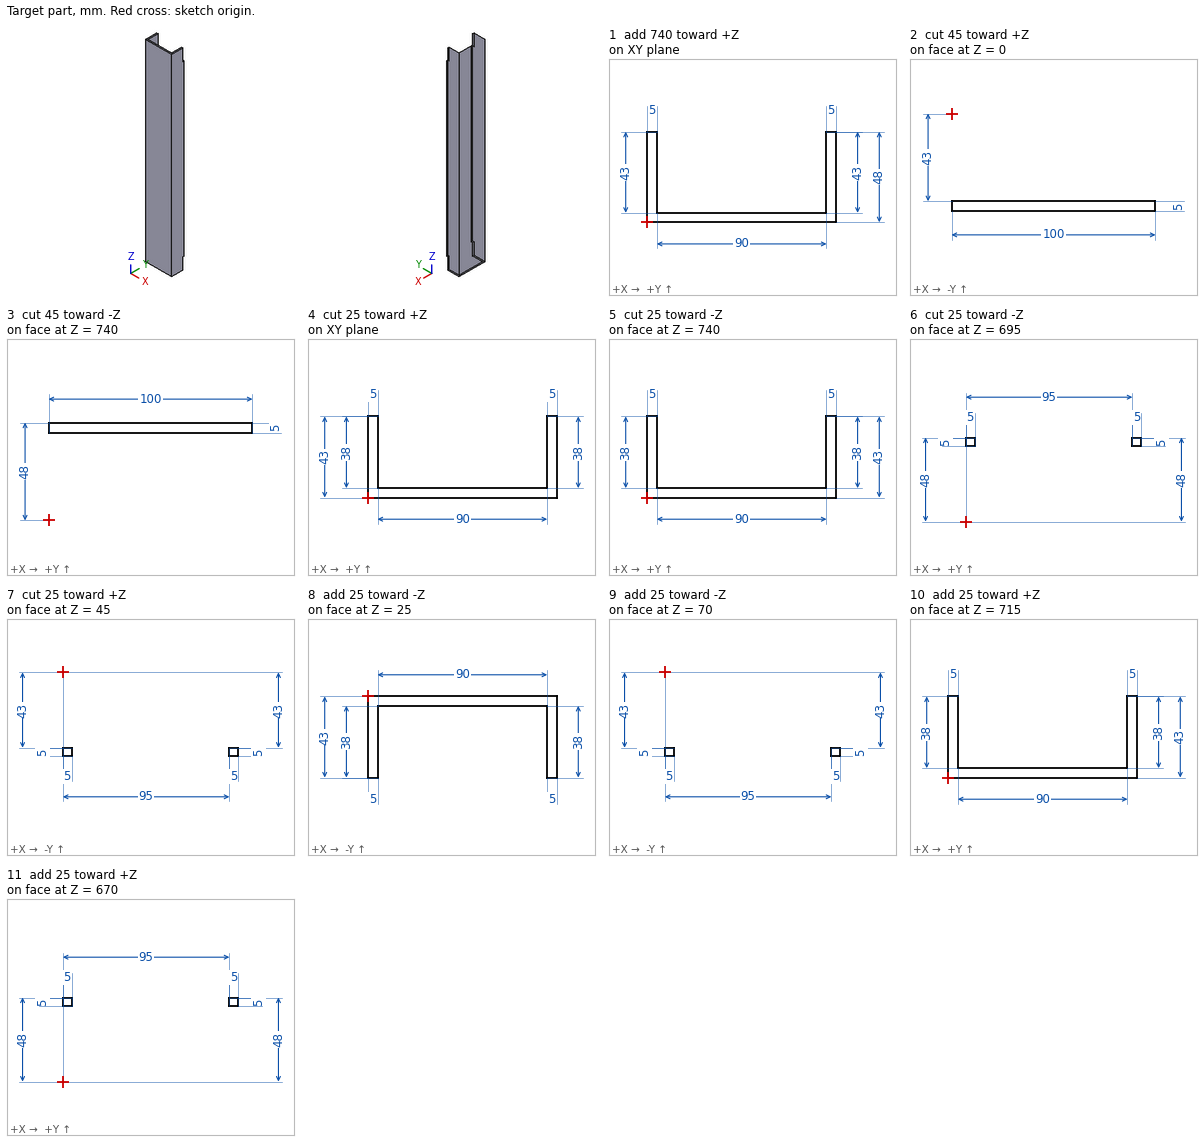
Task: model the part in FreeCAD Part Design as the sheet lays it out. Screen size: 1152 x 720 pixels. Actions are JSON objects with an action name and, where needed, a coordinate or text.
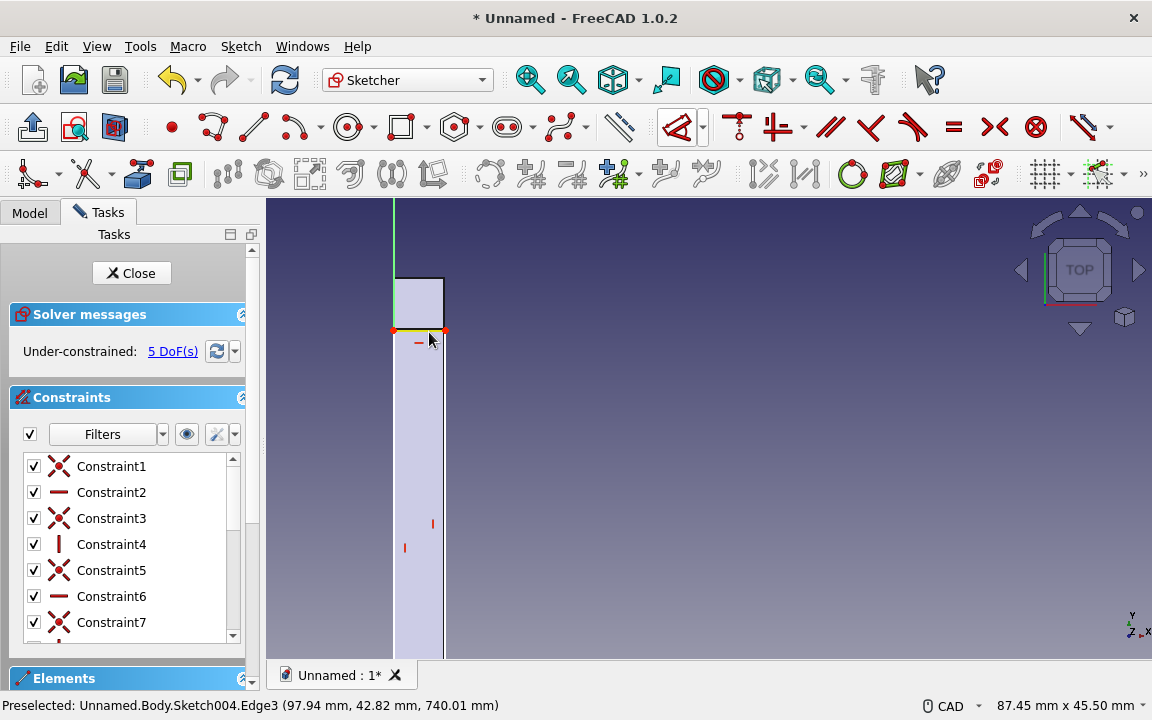
{"action": "left_click", "coordinate": [430, 331]}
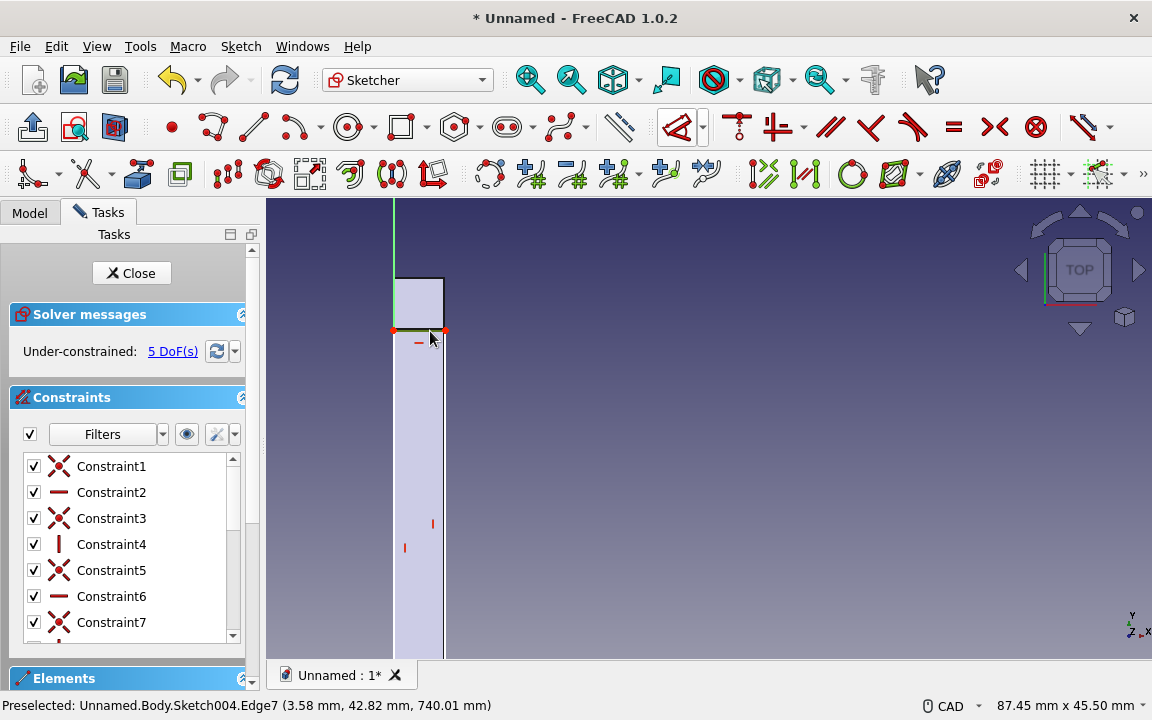
{"action": "left_click", "coordinate": [702, 128]}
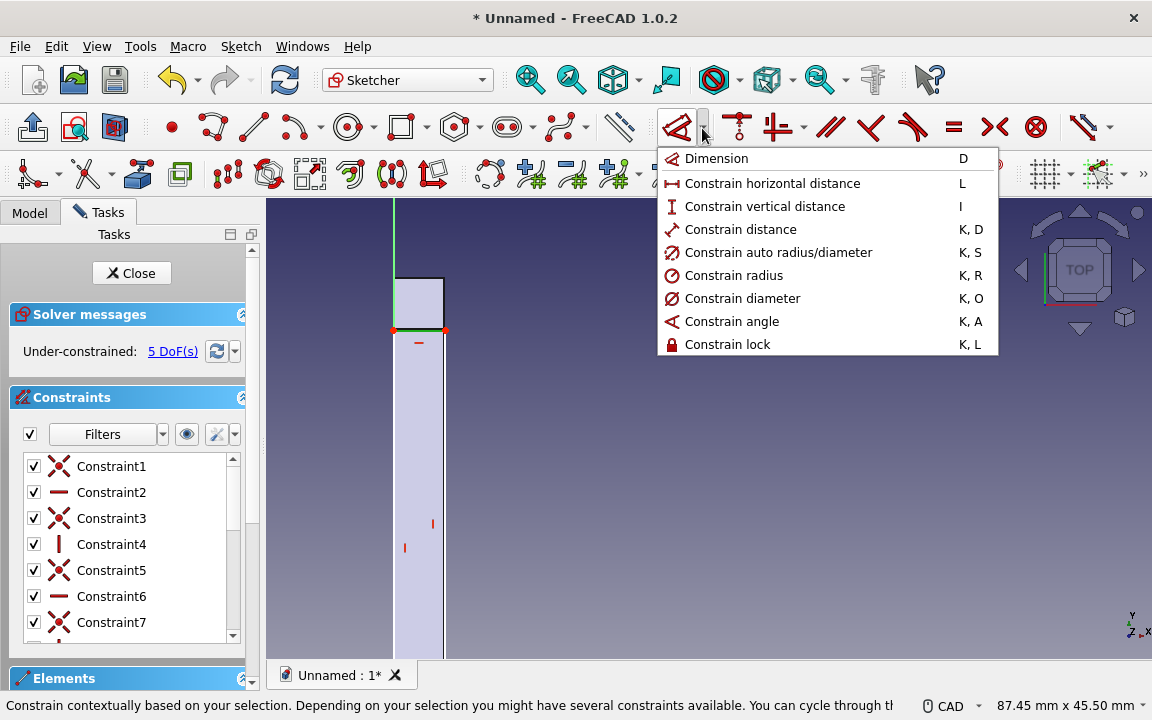
{"action": "left_click", "coordinate": [828, 184]}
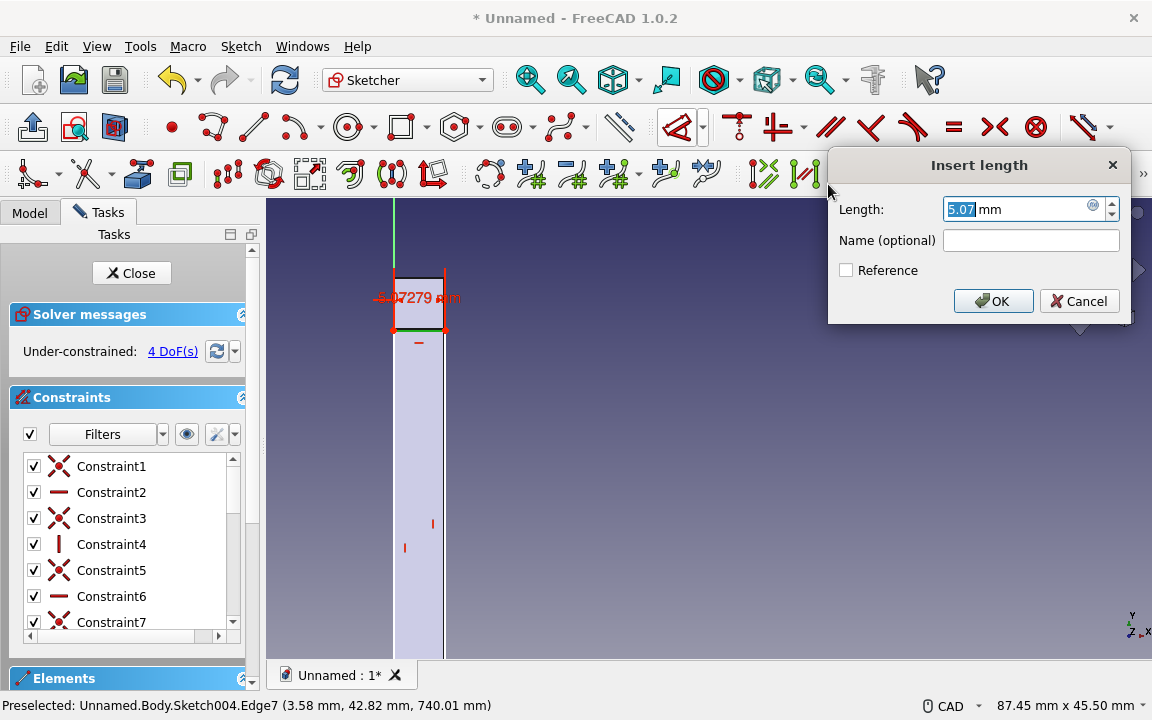
{"action": "type", "text": "5"}
{"action": "key", "text": "Return"}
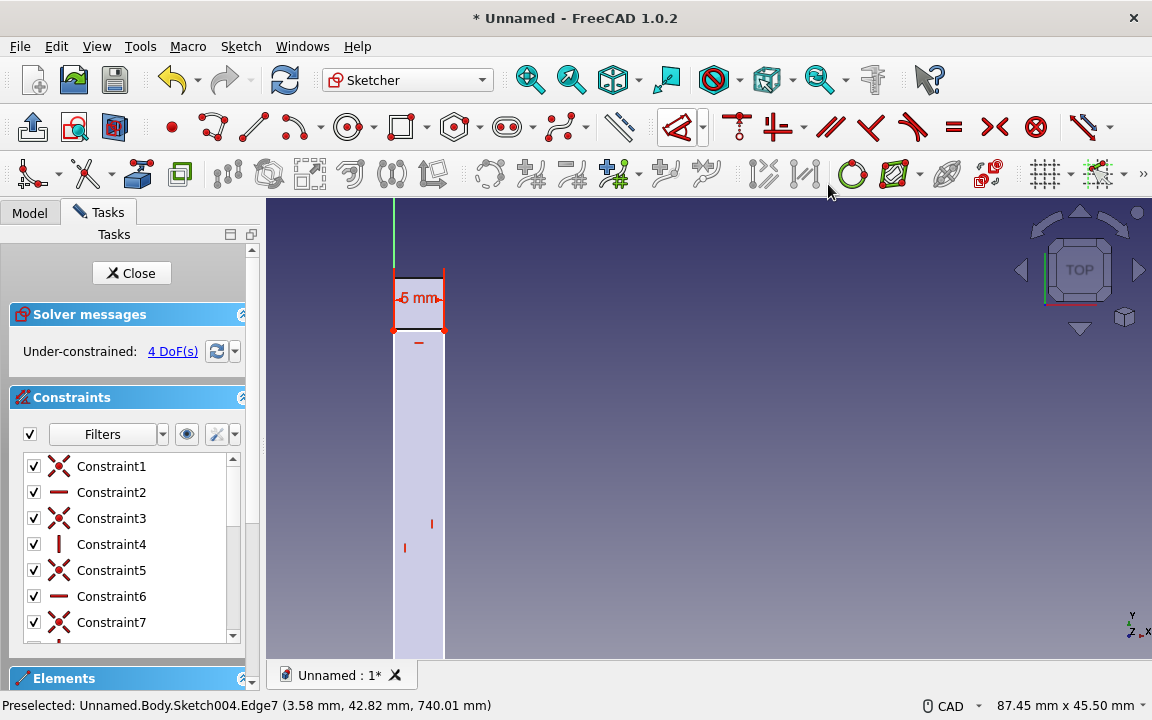
{"action": "scroll", "coordinate": [428, 332], "scroll_direction": "down", "scroll_amount": 4}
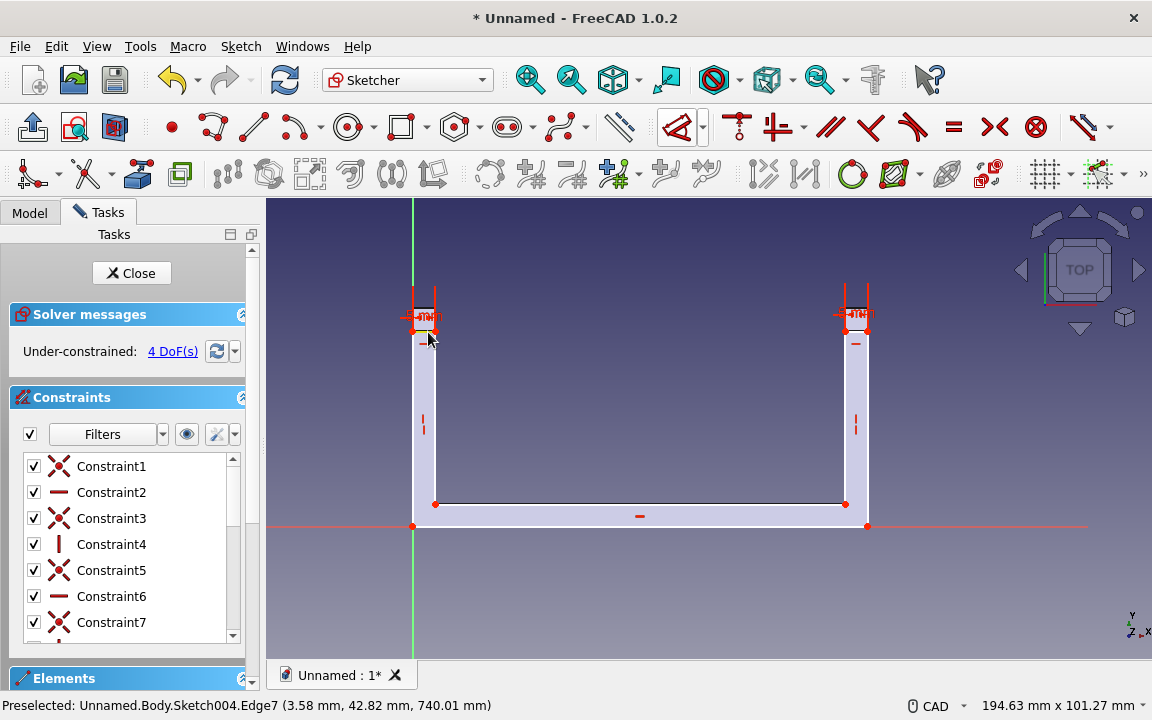
{"action": "left_click", "coordinate": [868, 468]}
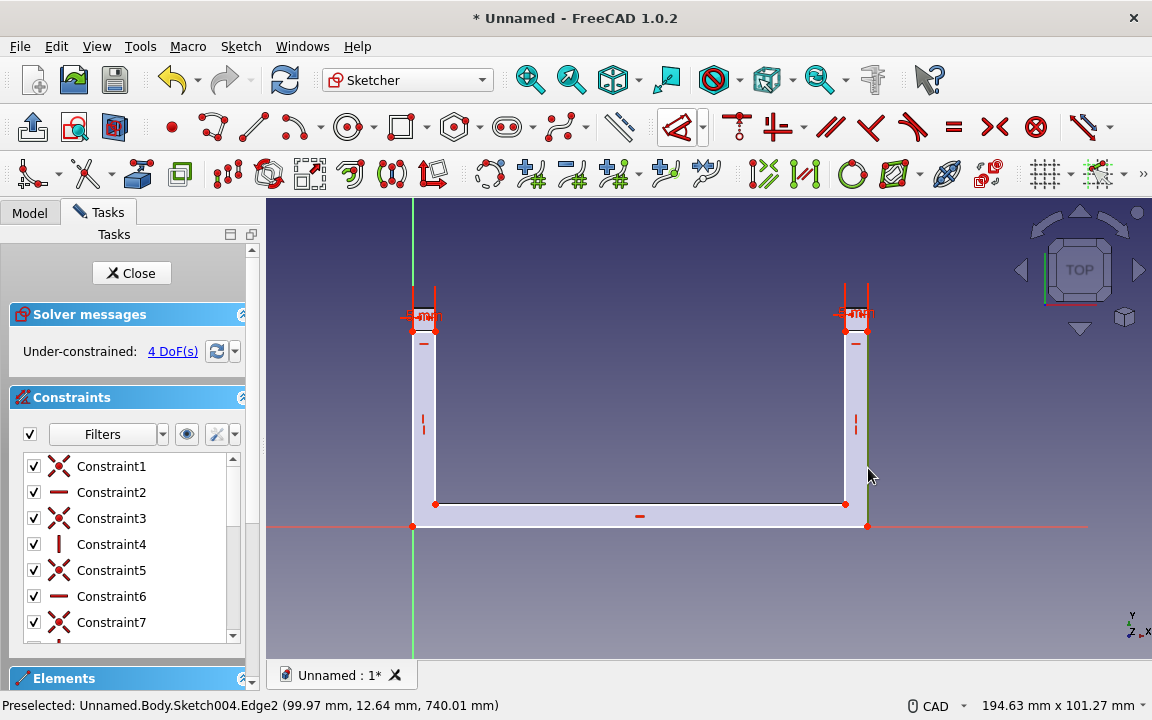
{"action": "key", "text": "i"}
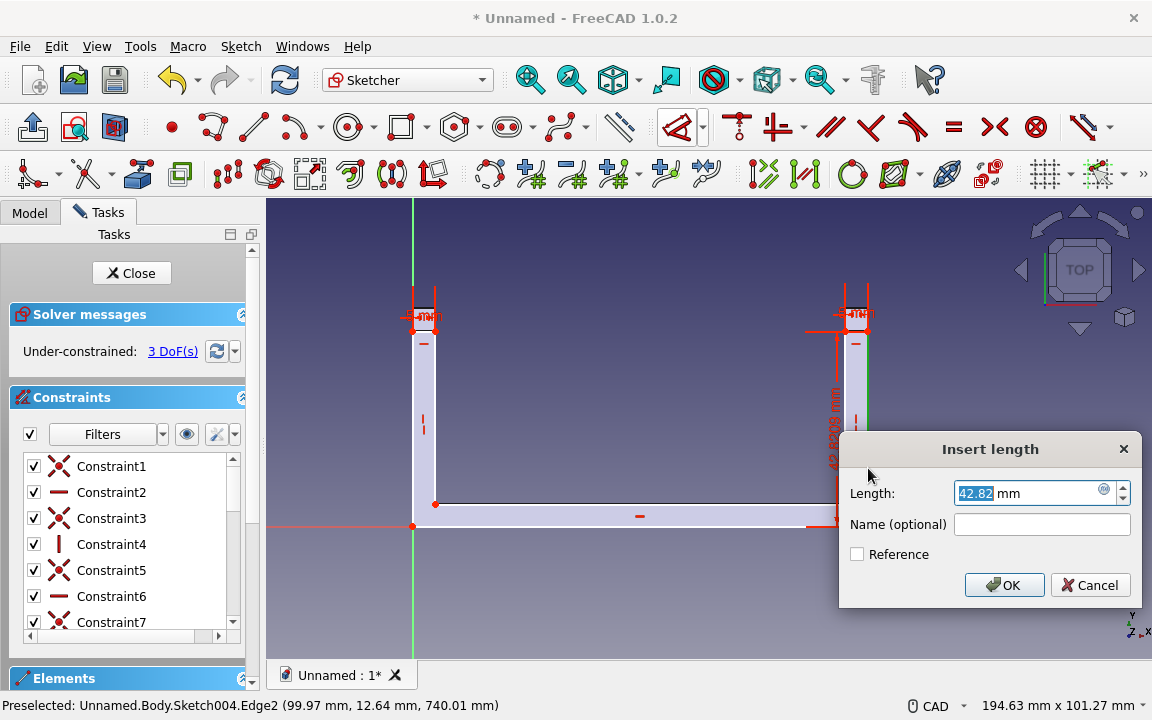
{"action": "type", "text": "43"}
{"action": "key", "text": "Return"}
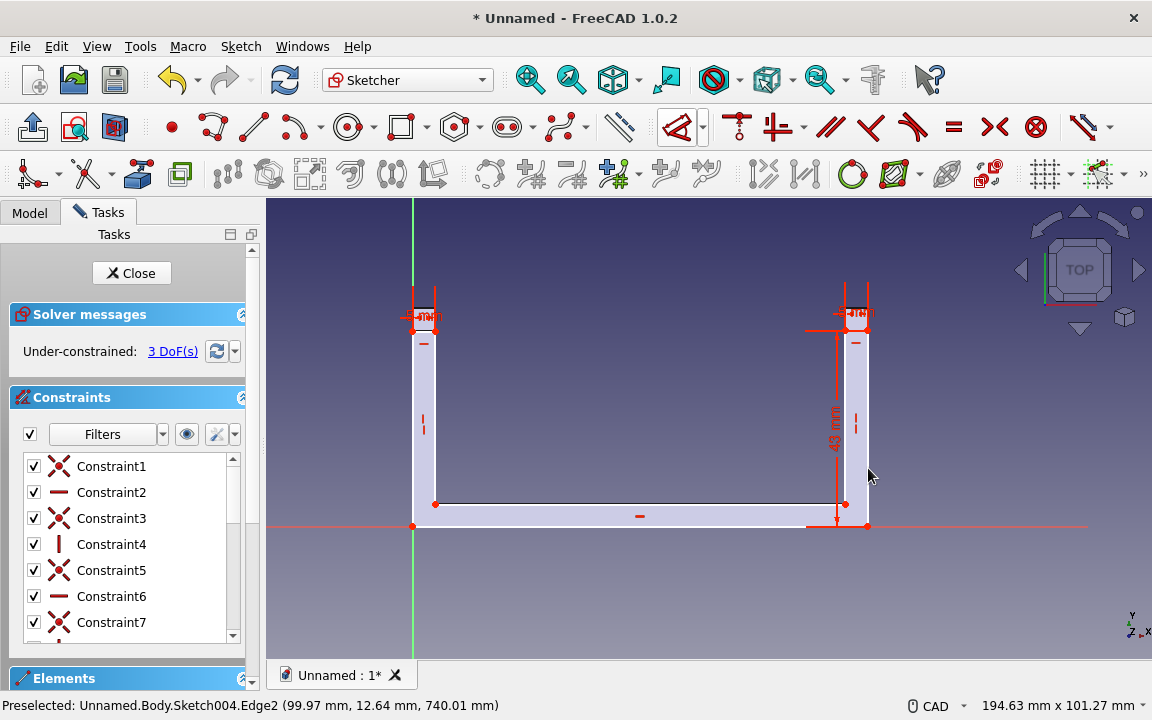
{"action": "left_click", "coordinate": [845, 383]}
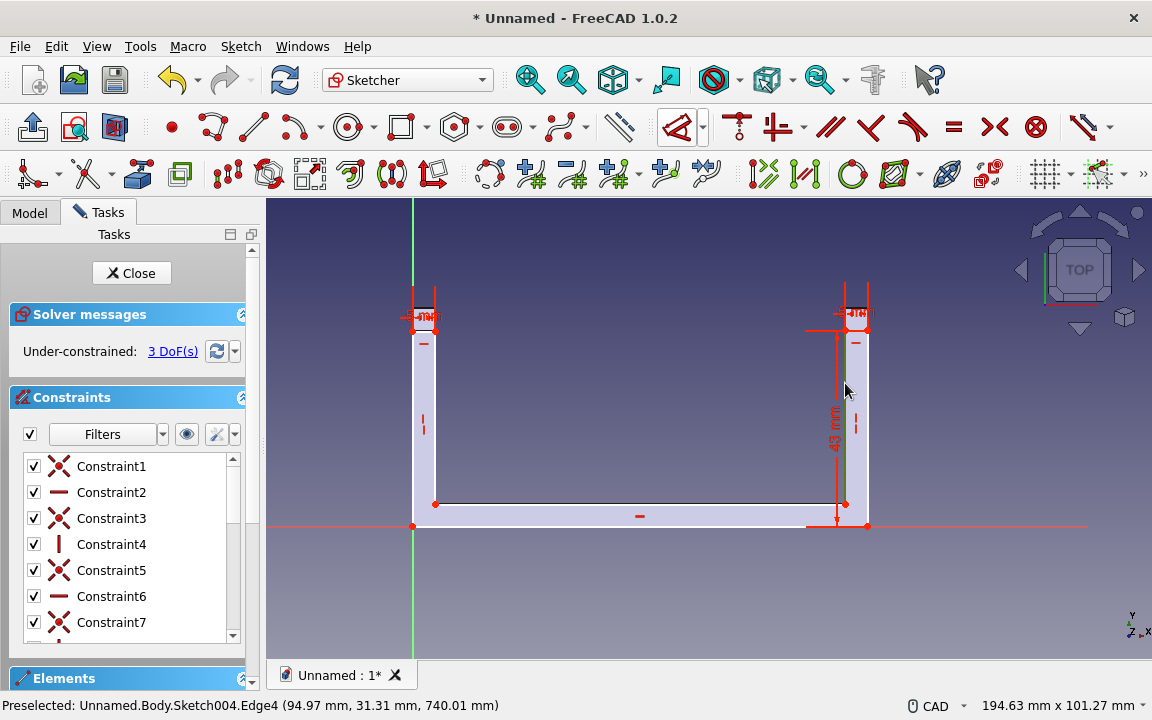
{"action": "left_click", "coordinate": [702, 128]}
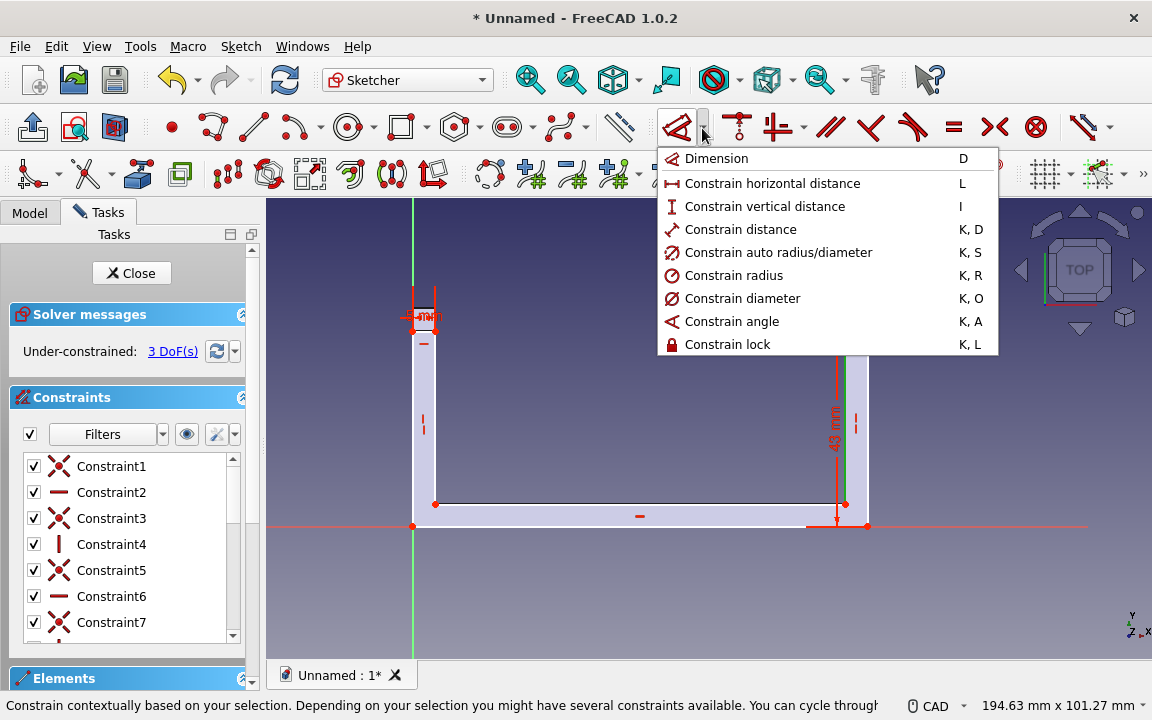
{"action": "left_click", "coordinate": [828, 206]}